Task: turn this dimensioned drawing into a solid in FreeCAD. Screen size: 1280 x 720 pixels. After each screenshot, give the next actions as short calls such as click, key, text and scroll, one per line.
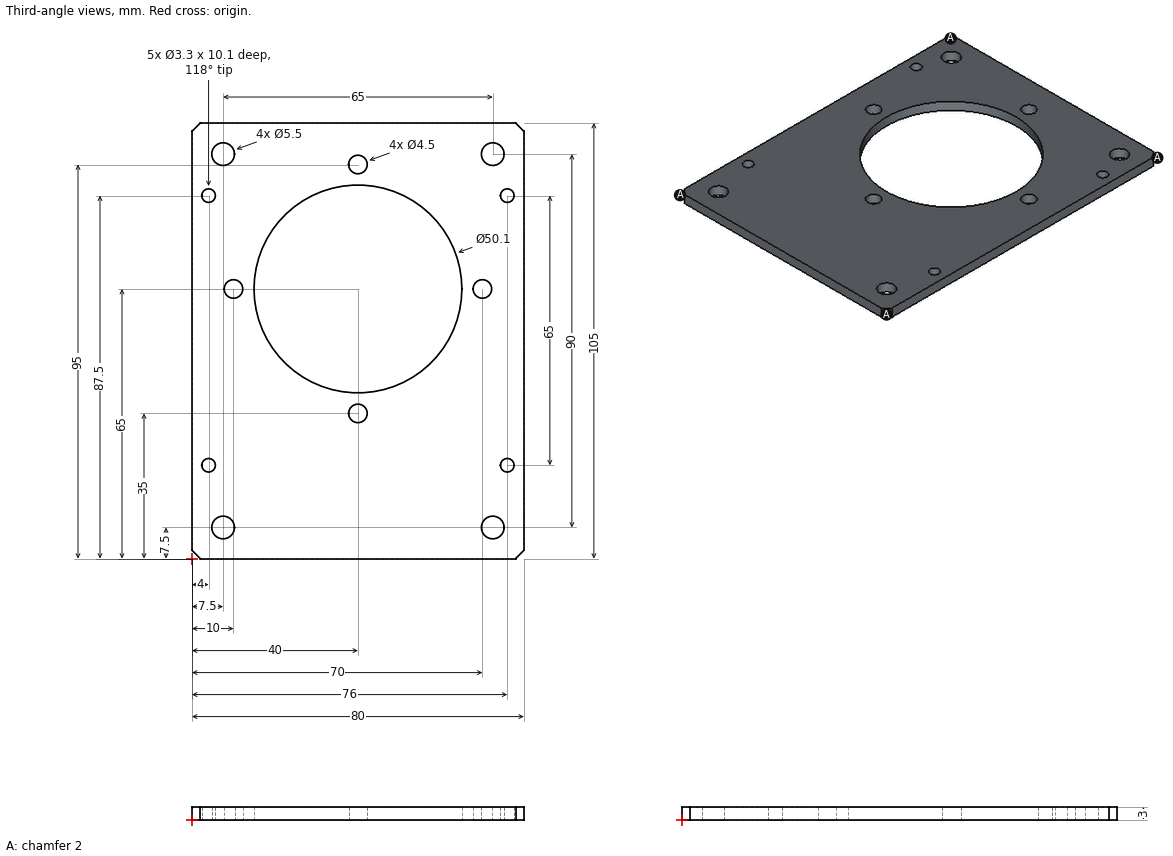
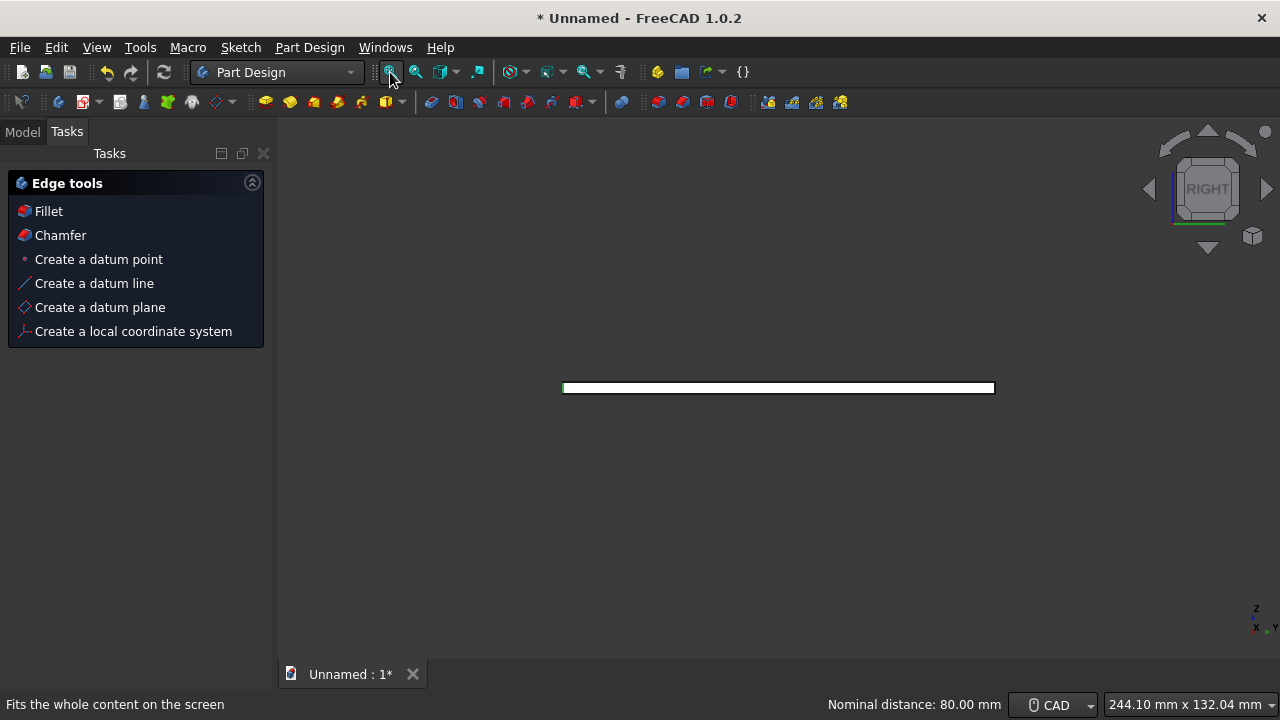
click(995, 387, ctrl)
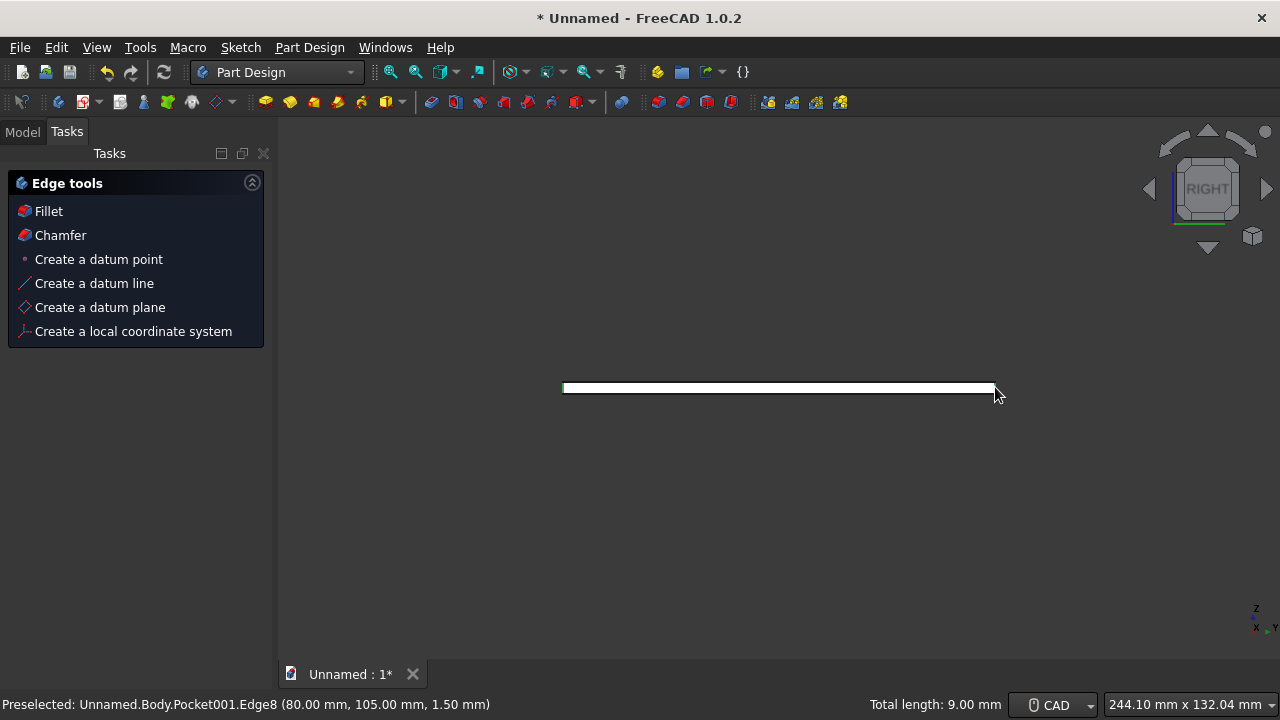
scroll(995, 387, up, 6)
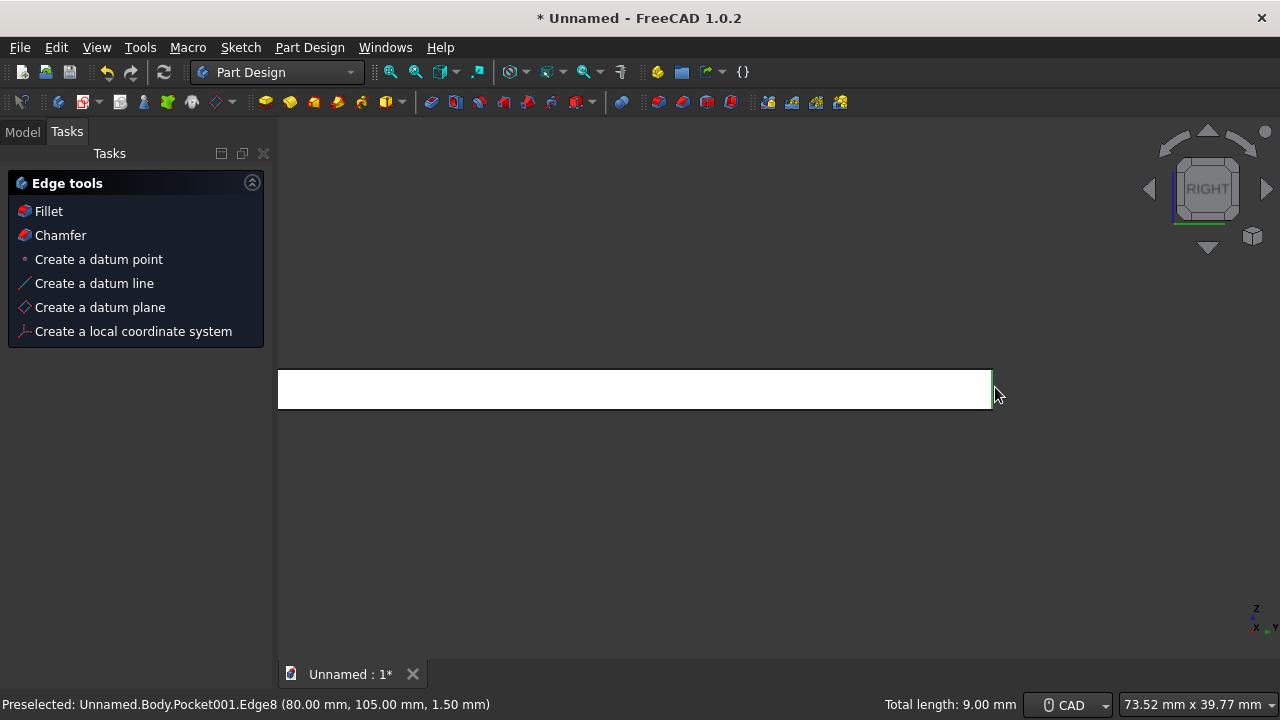
click(392, 72)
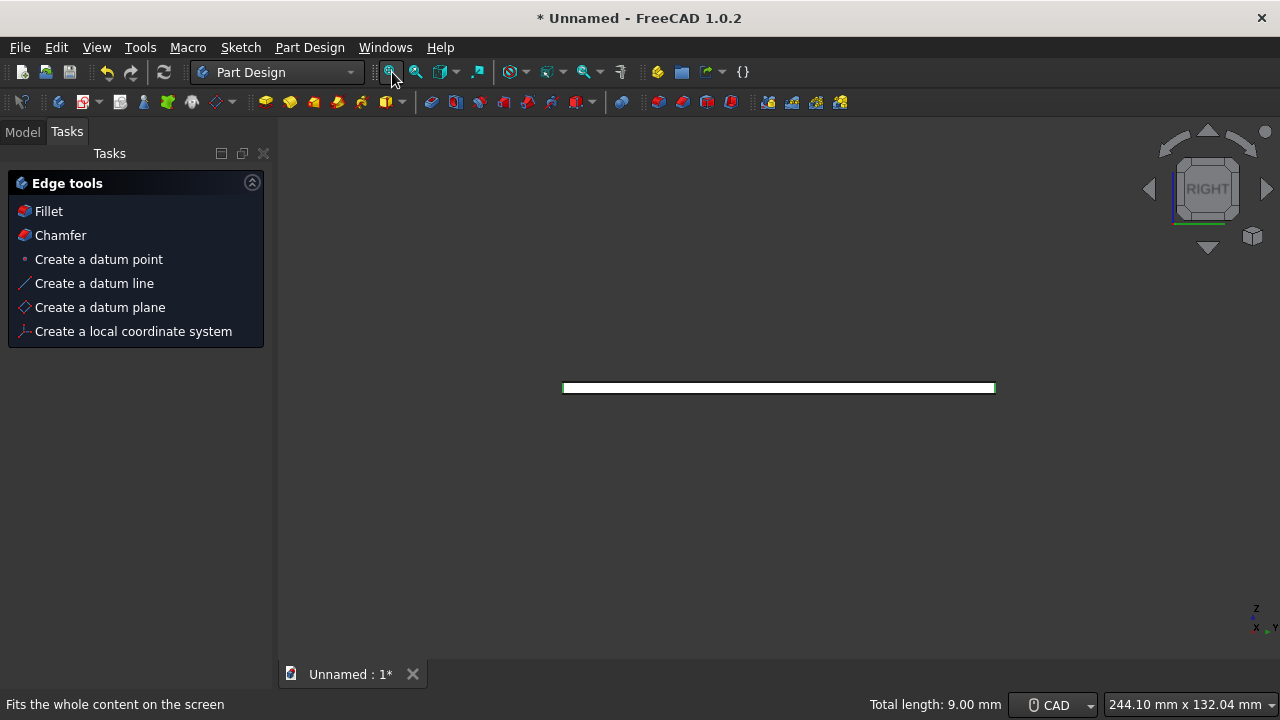
key(5)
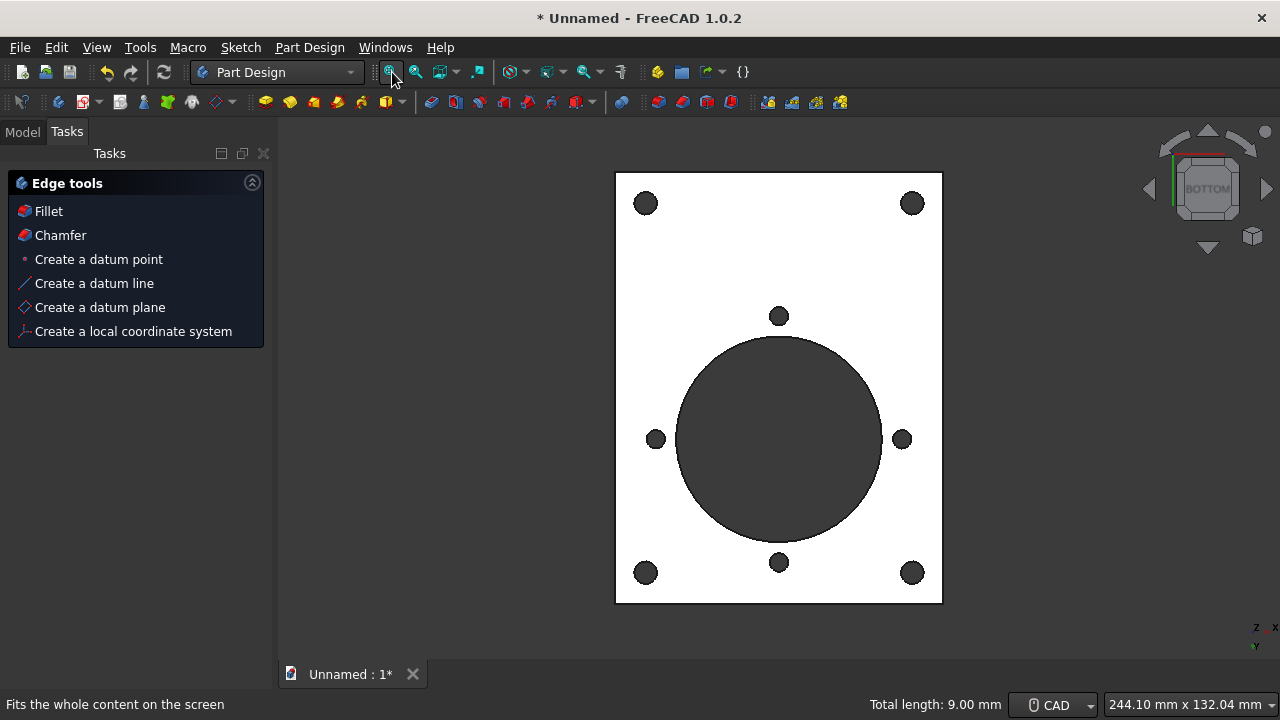
scroll(615, 603, up, 6)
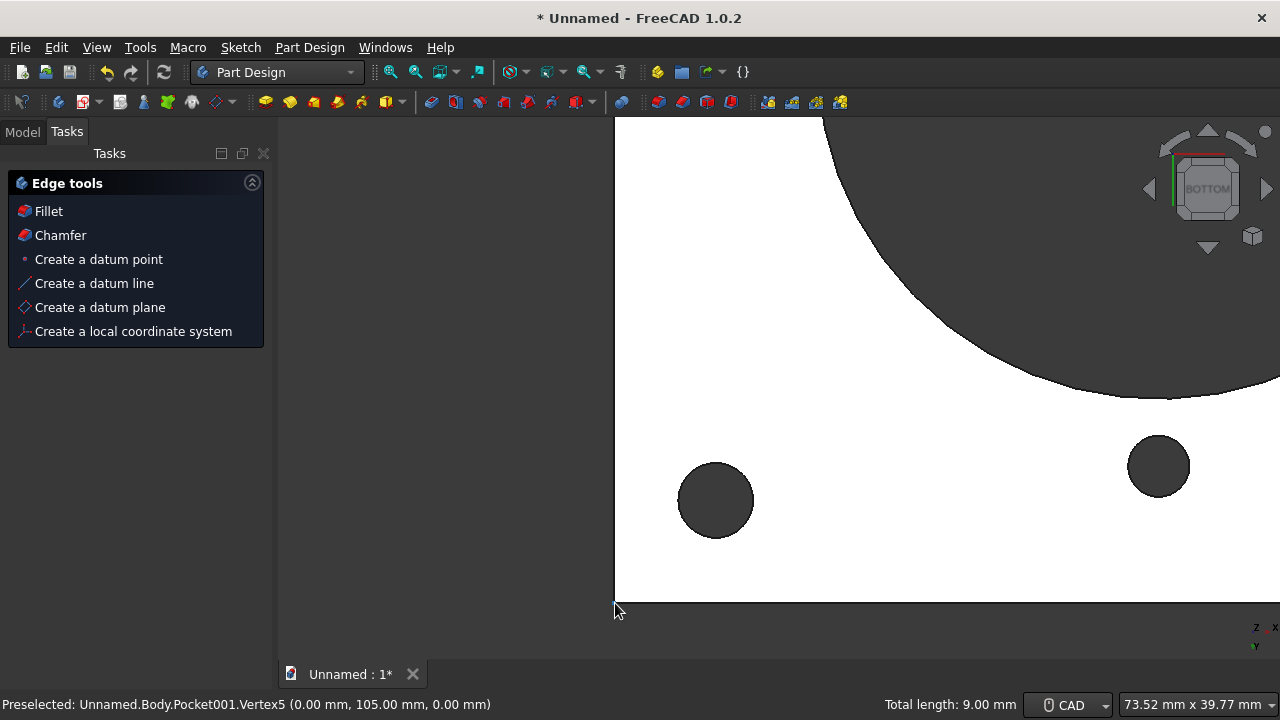
click(392, 72)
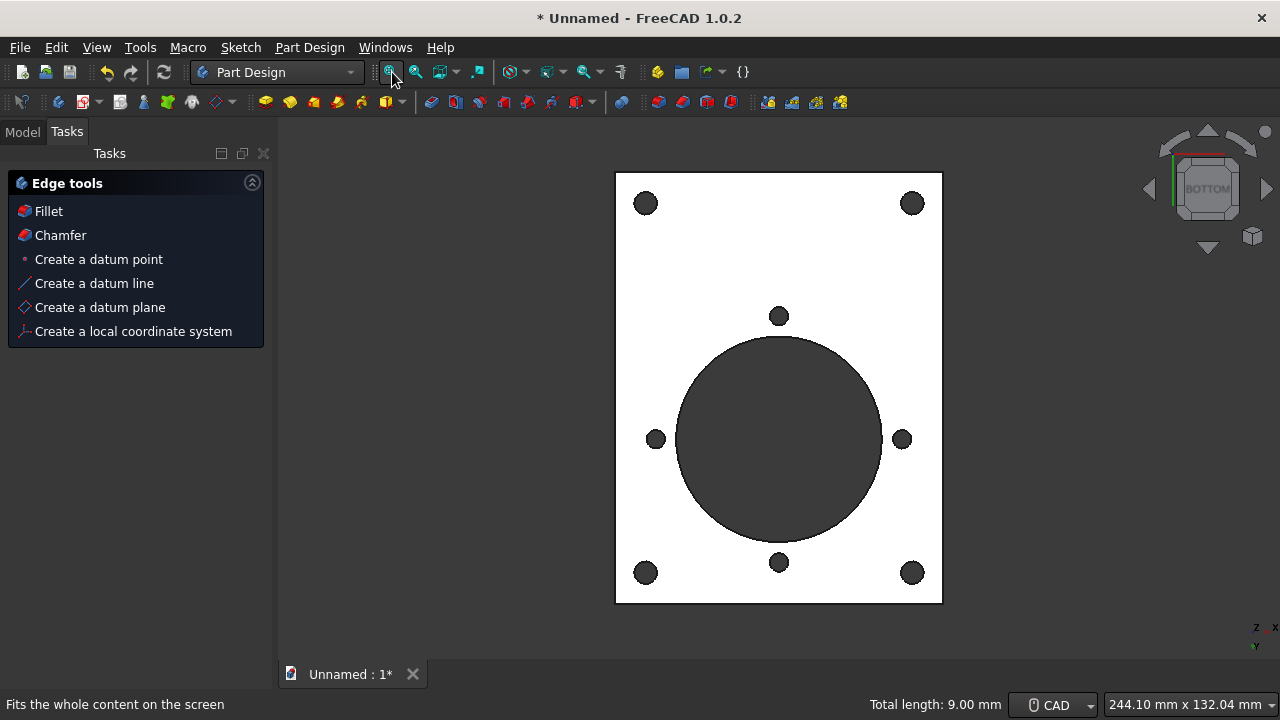
key(4)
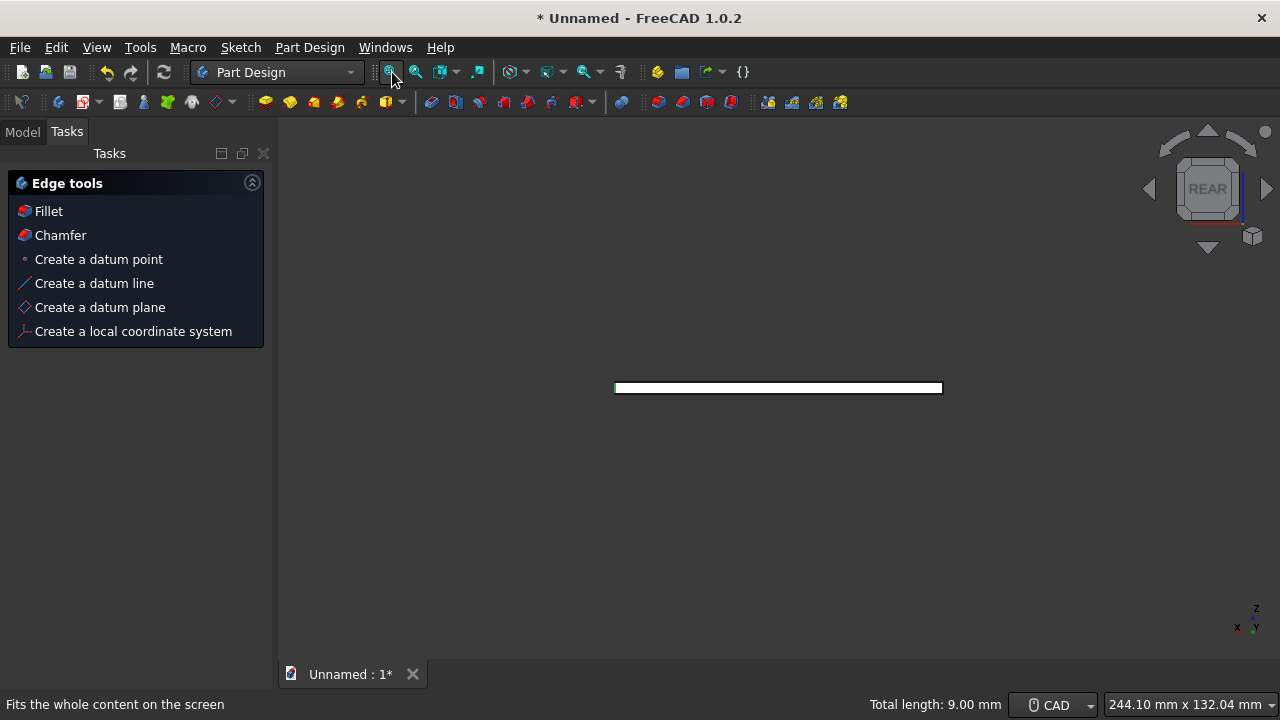
key(v)
key(f)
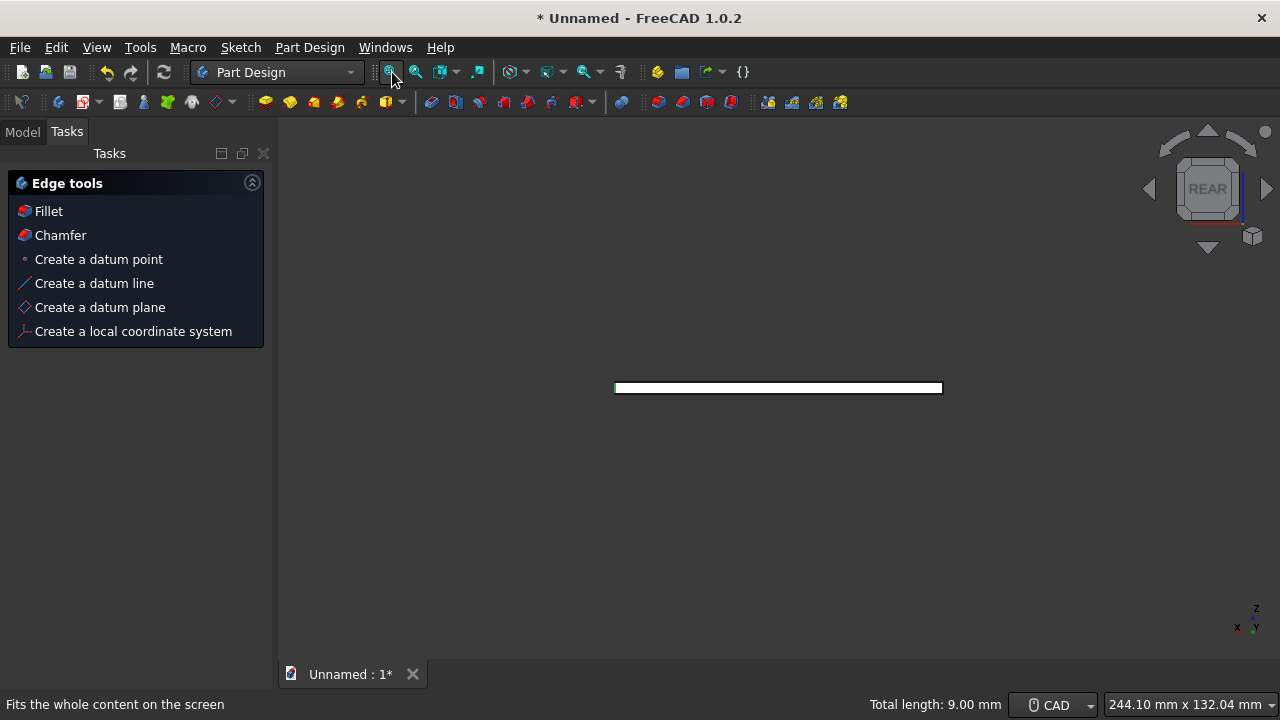
click(943, 387, ctrl)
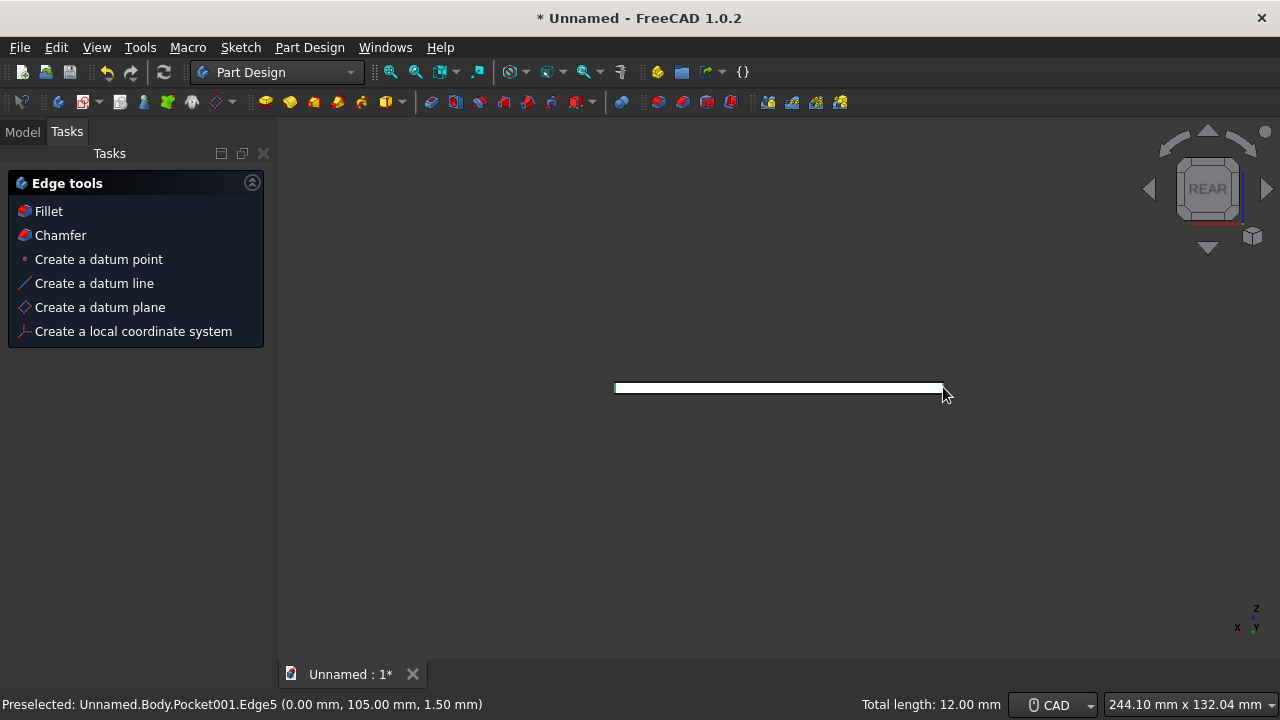
click(684, 102)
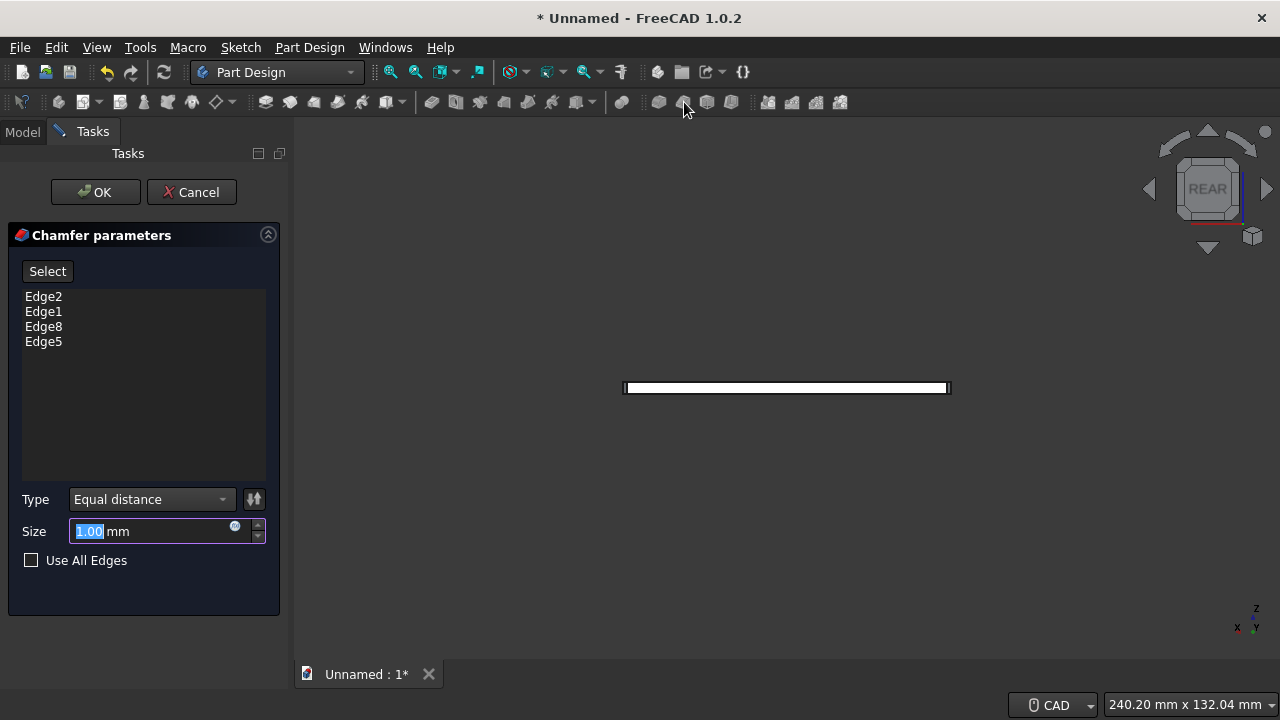
text(2)
key(Tab)